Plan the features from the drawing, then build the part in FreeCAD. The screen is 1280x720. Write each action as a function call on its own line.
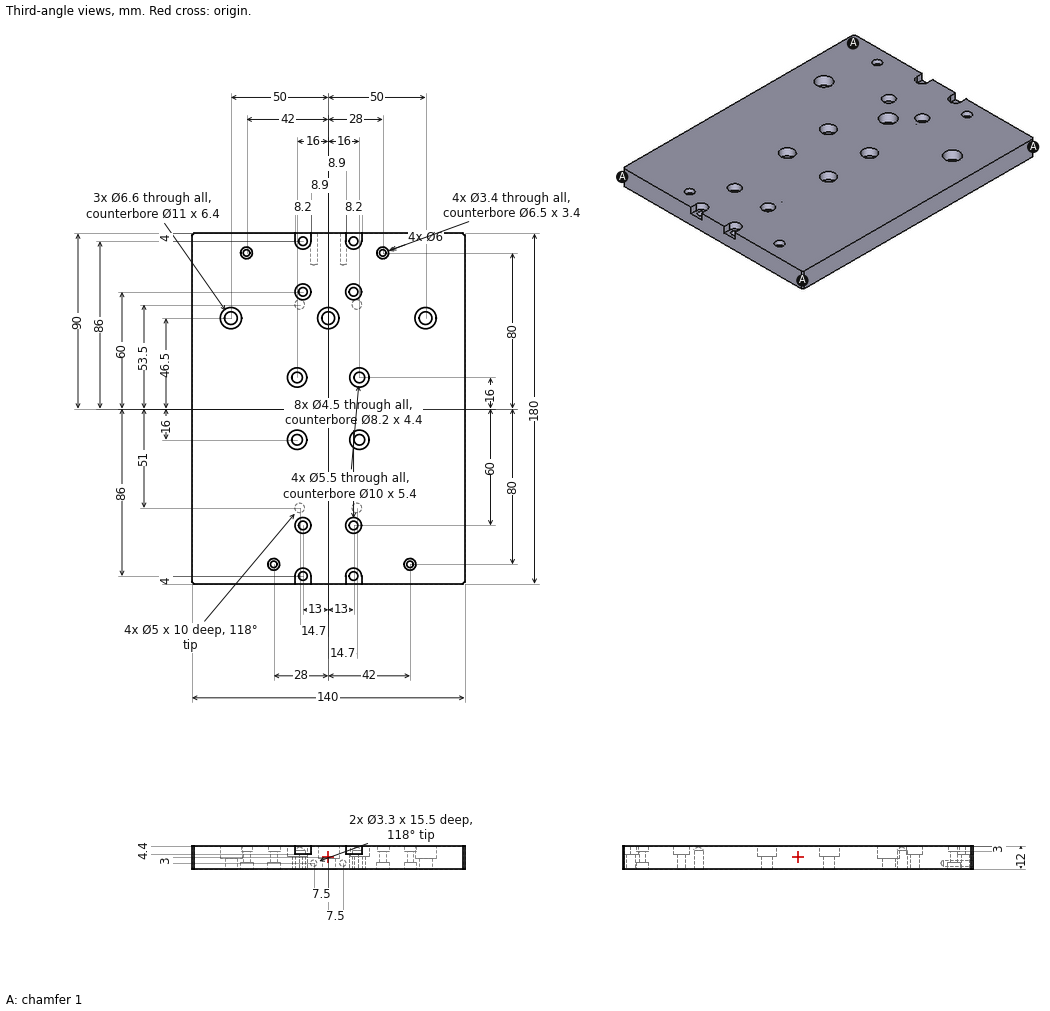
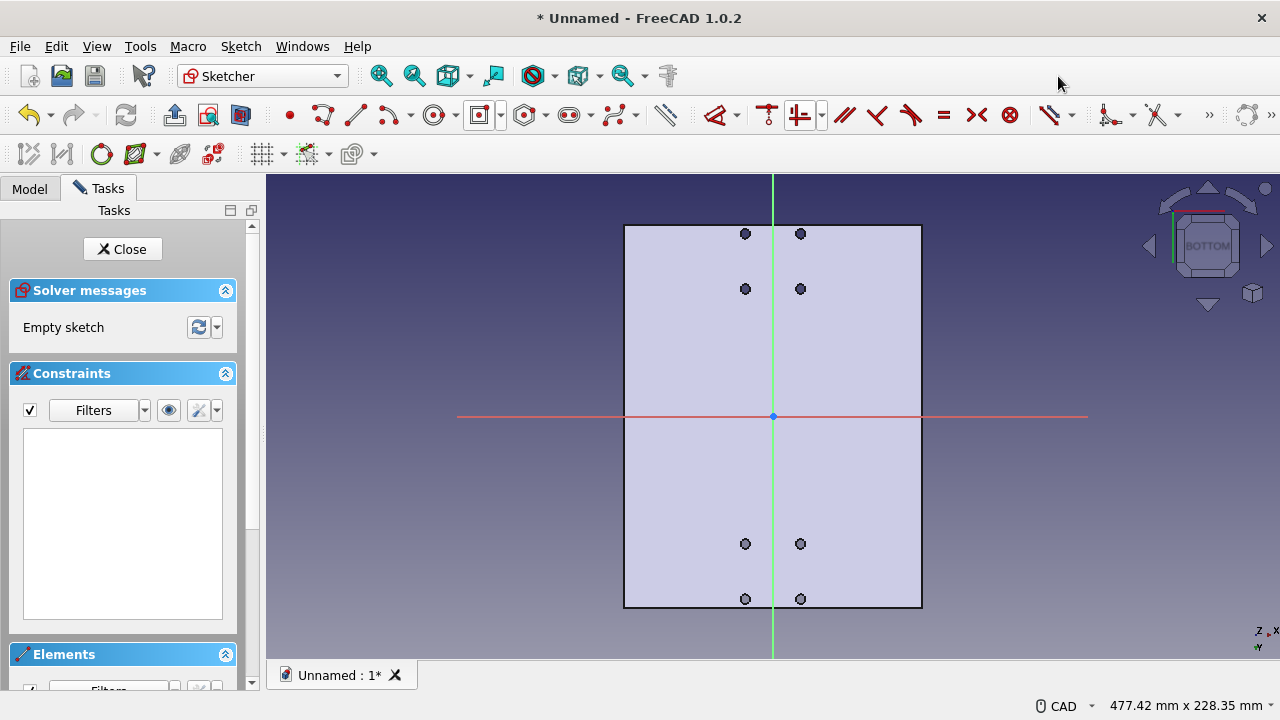
click(434, 116)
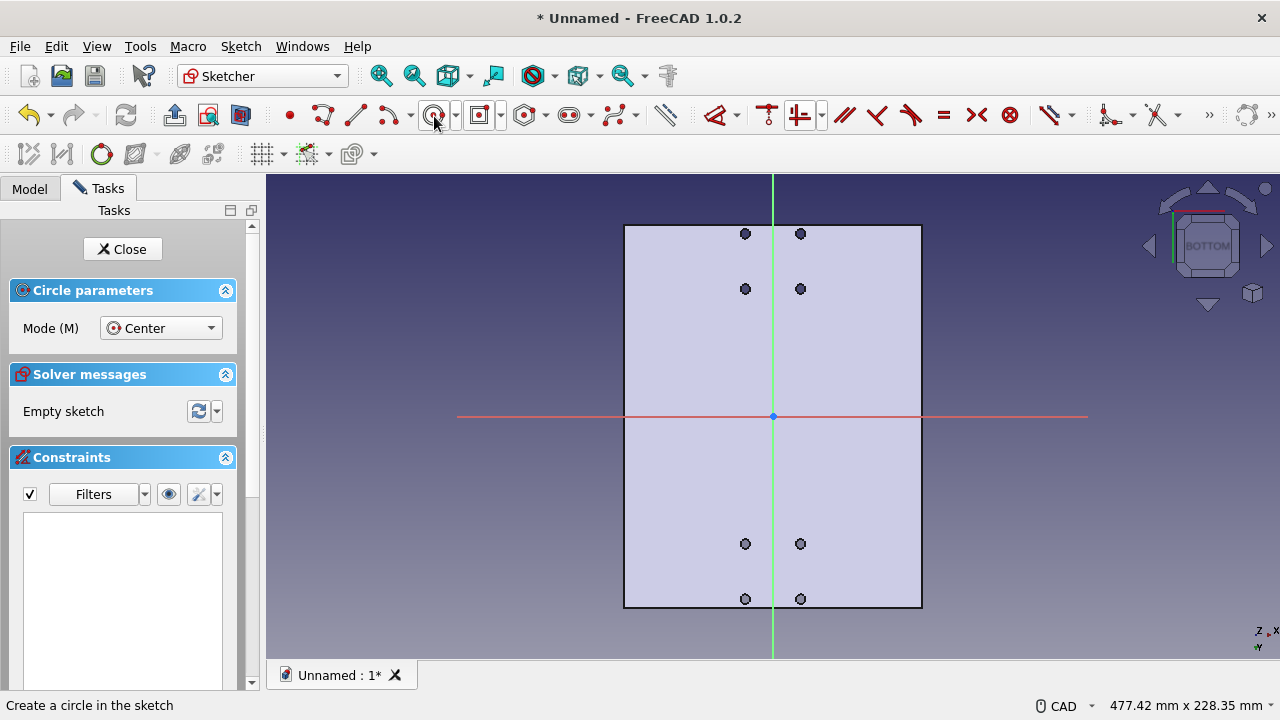
scroll(742, 308, up, 8)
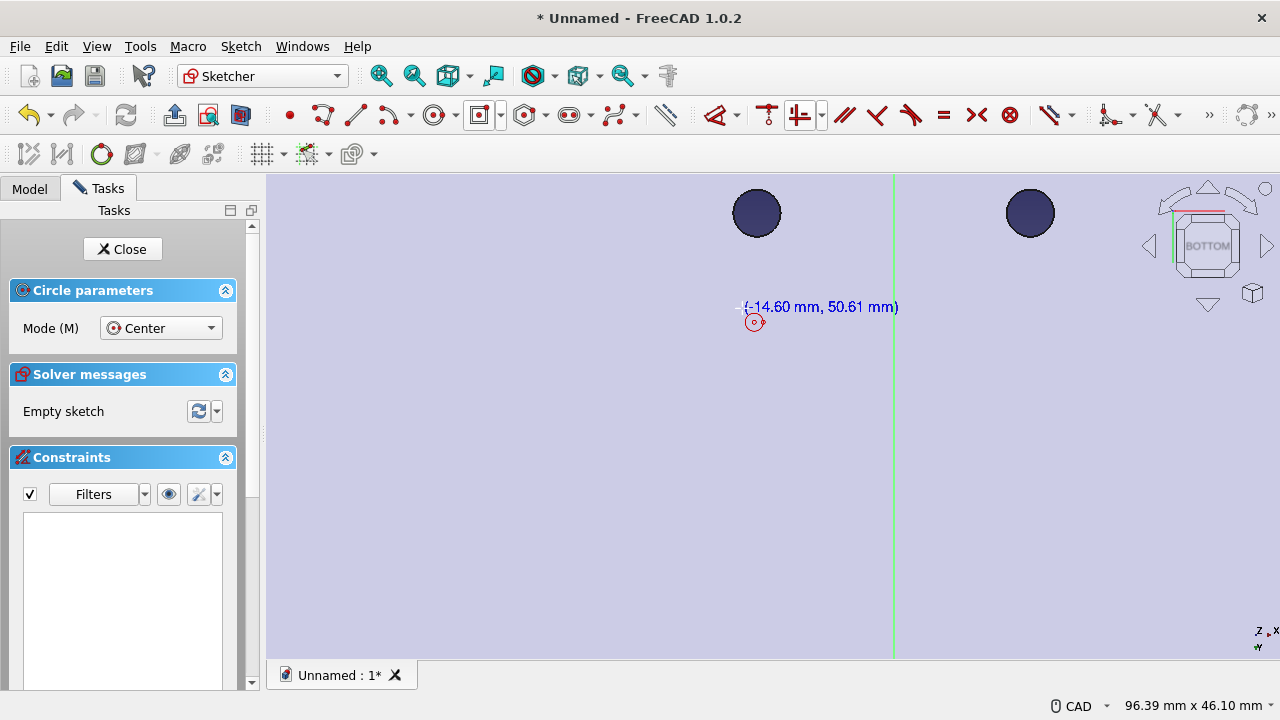
scroll(643, 272, down, 7)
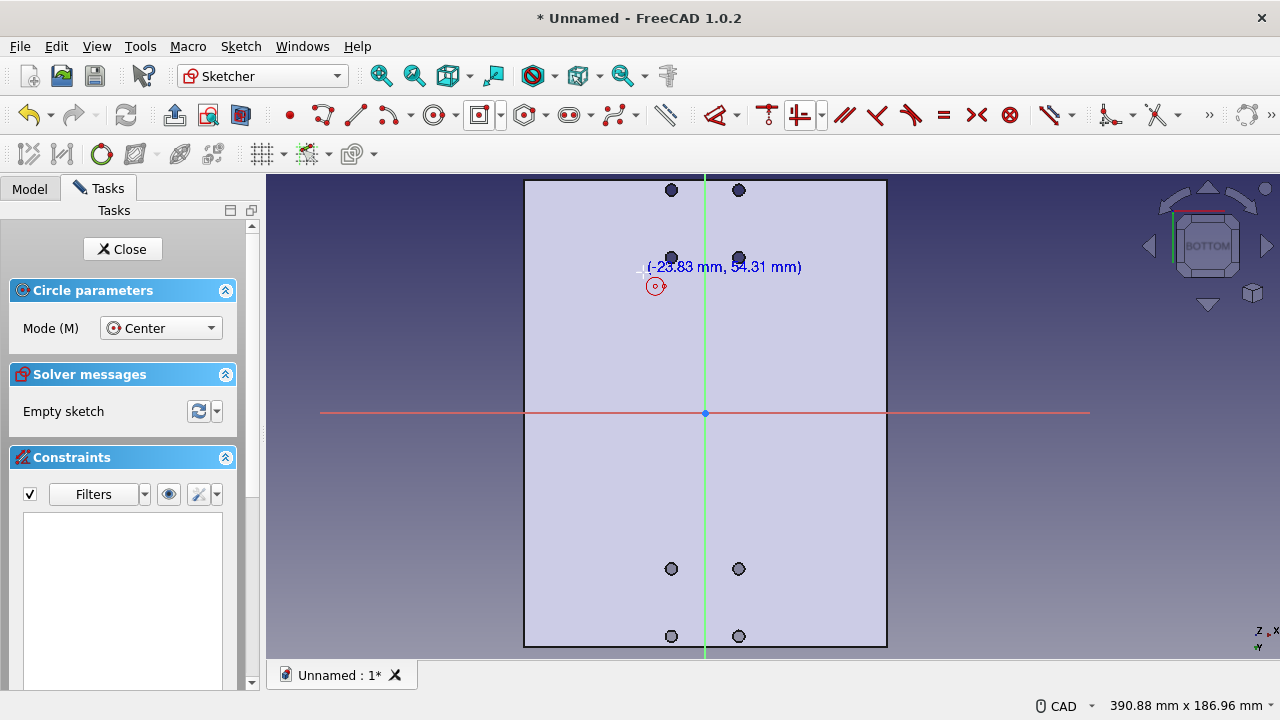
click(667, 281)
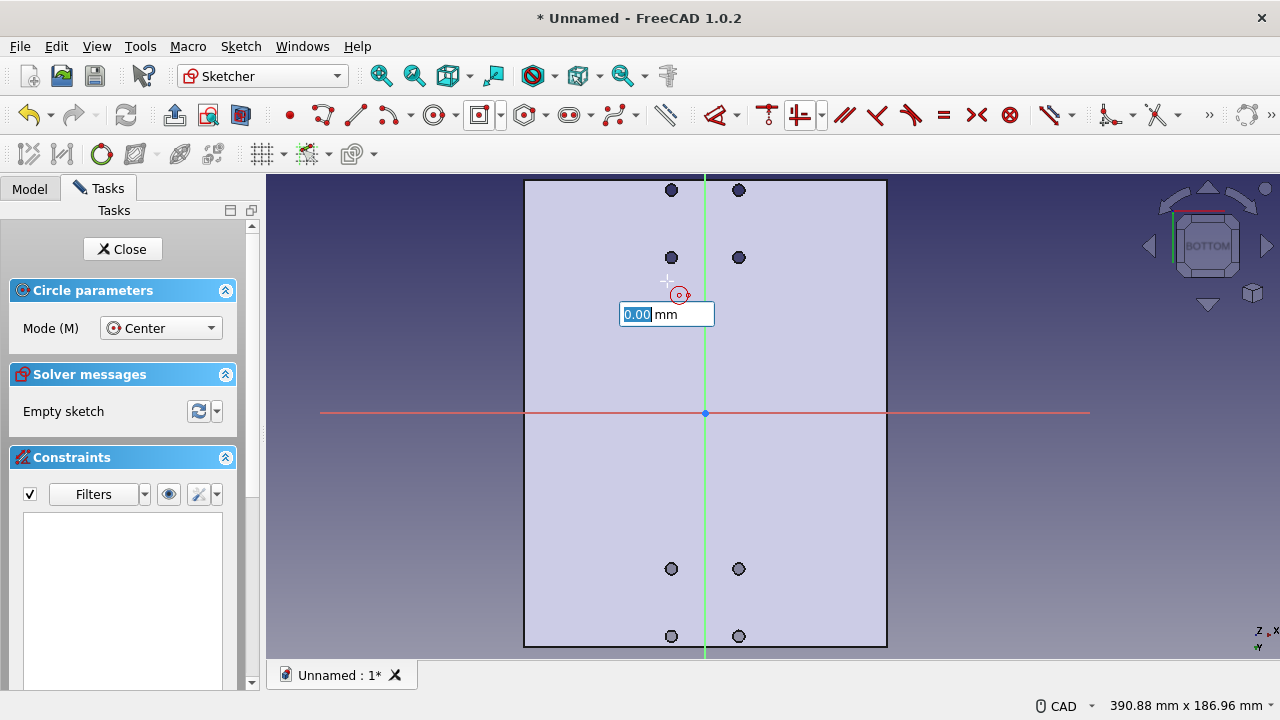
scroll(672, 276, up, 5)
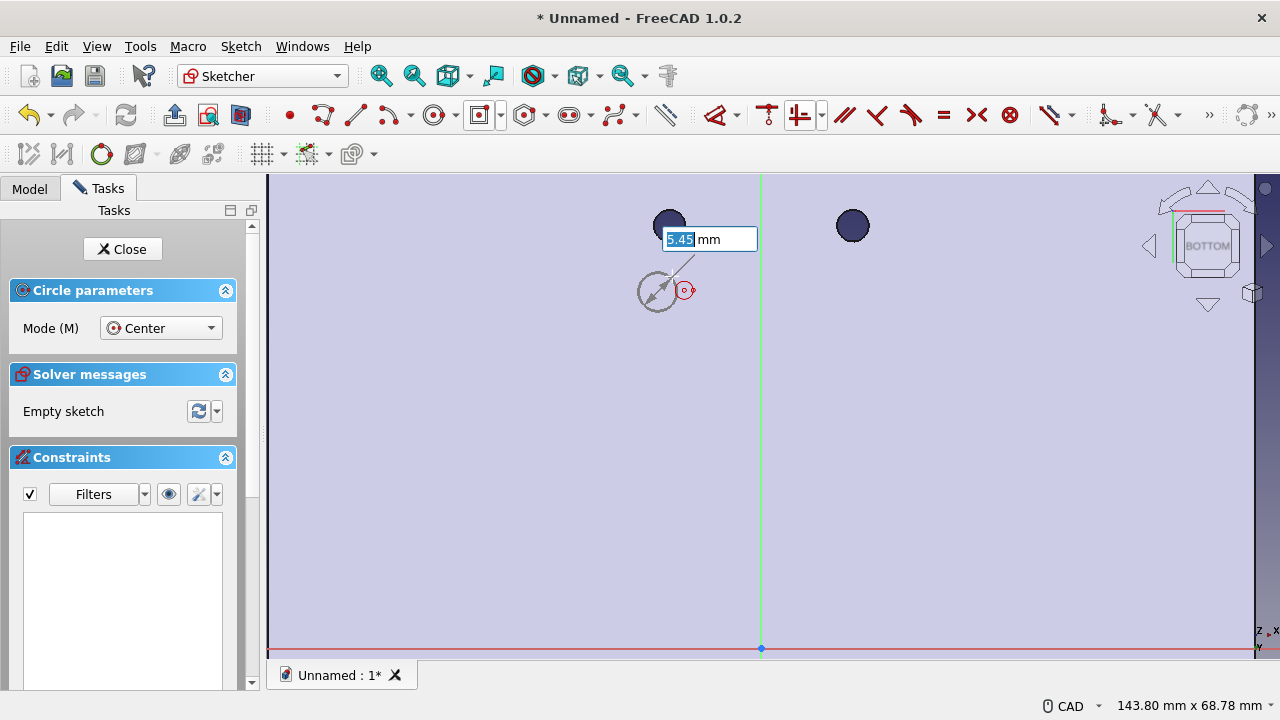
click(670, 277)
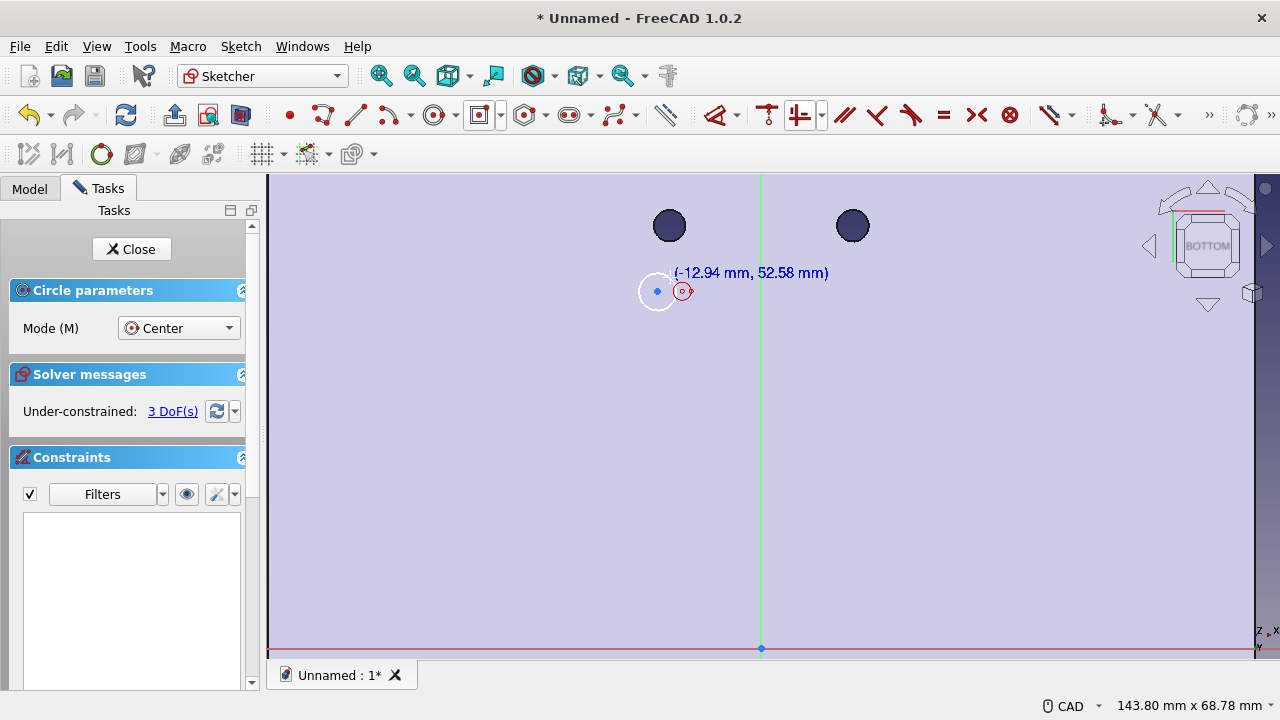
scroll(865, 289, up, 2)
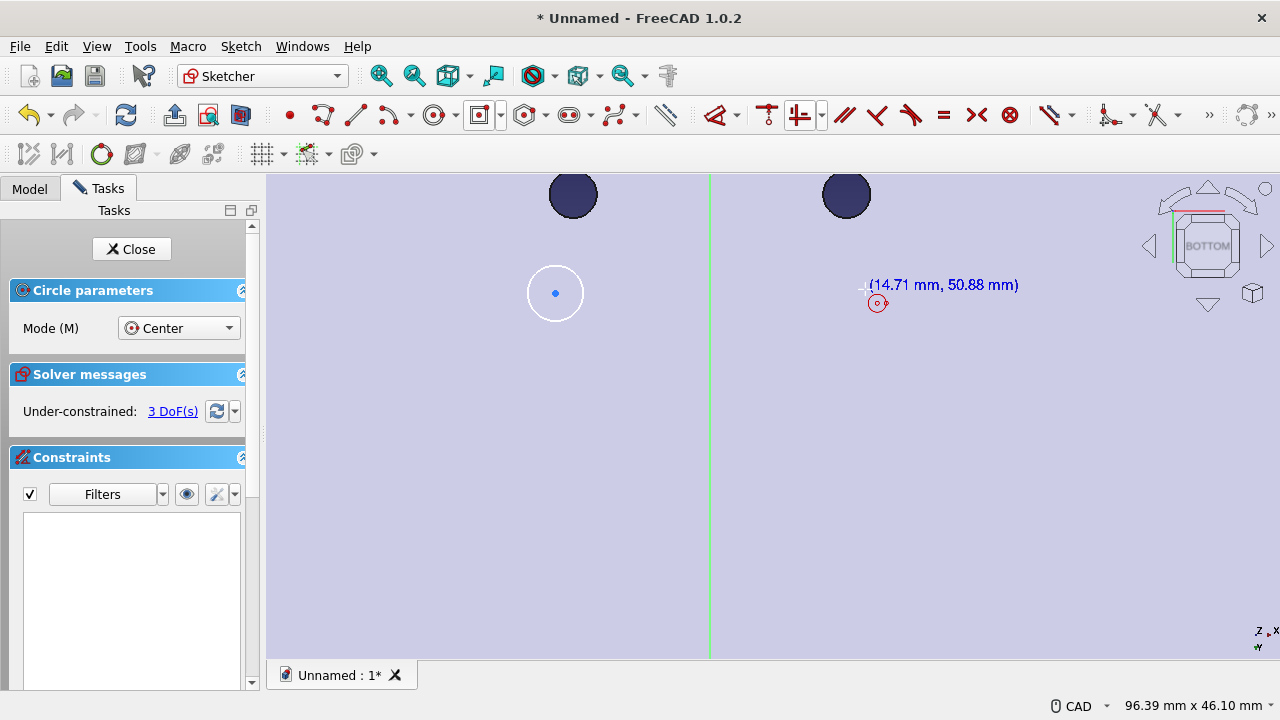
scroll(703, 278, down, 7)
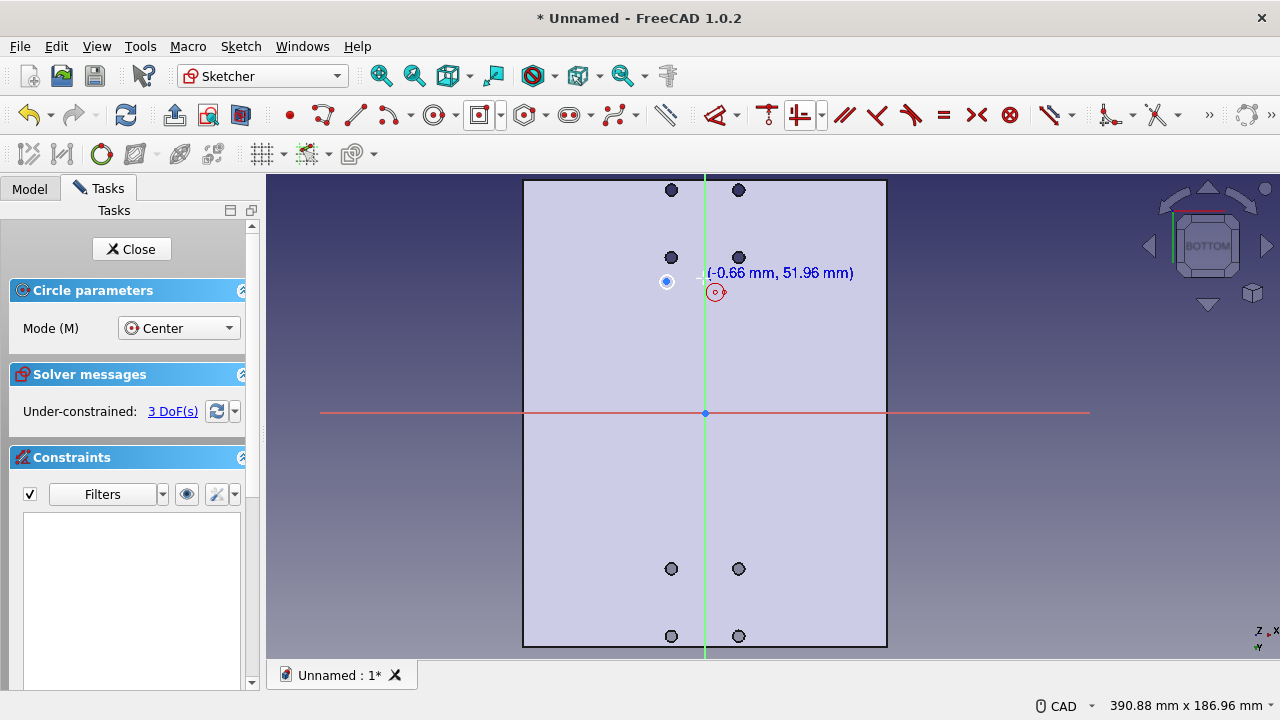
click(743, 281)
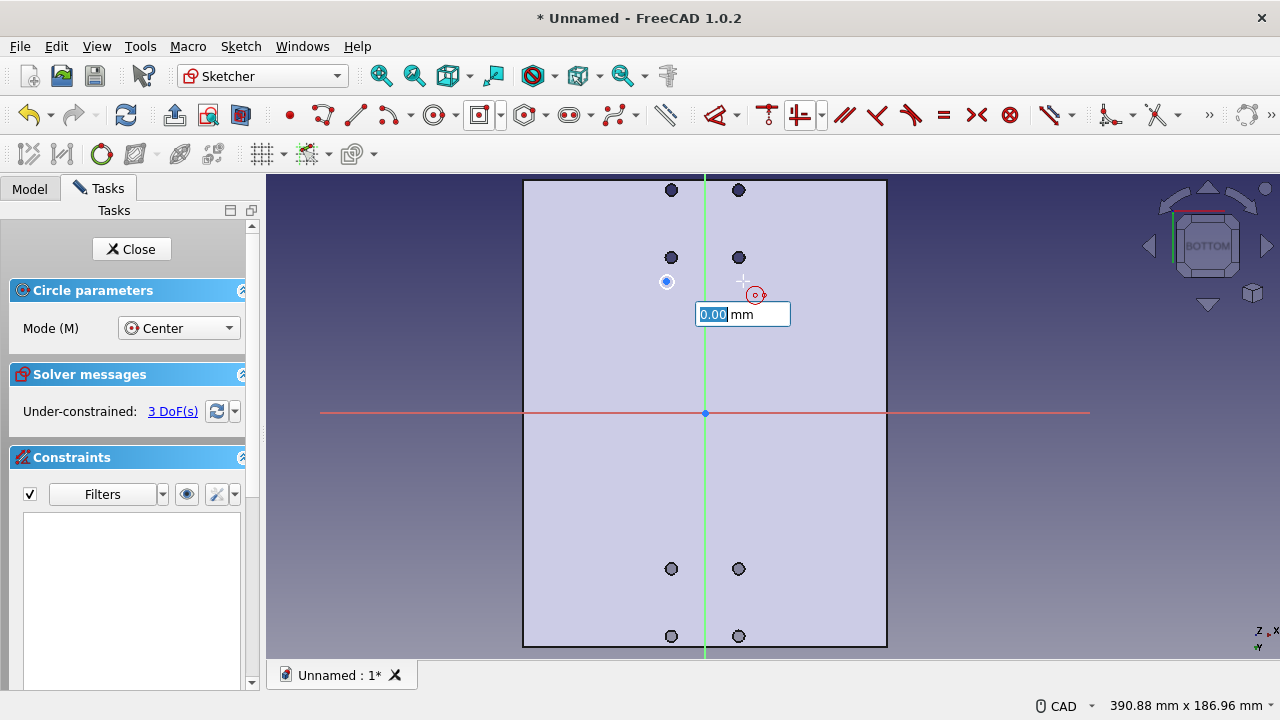
scroll(748, 276, up, 5)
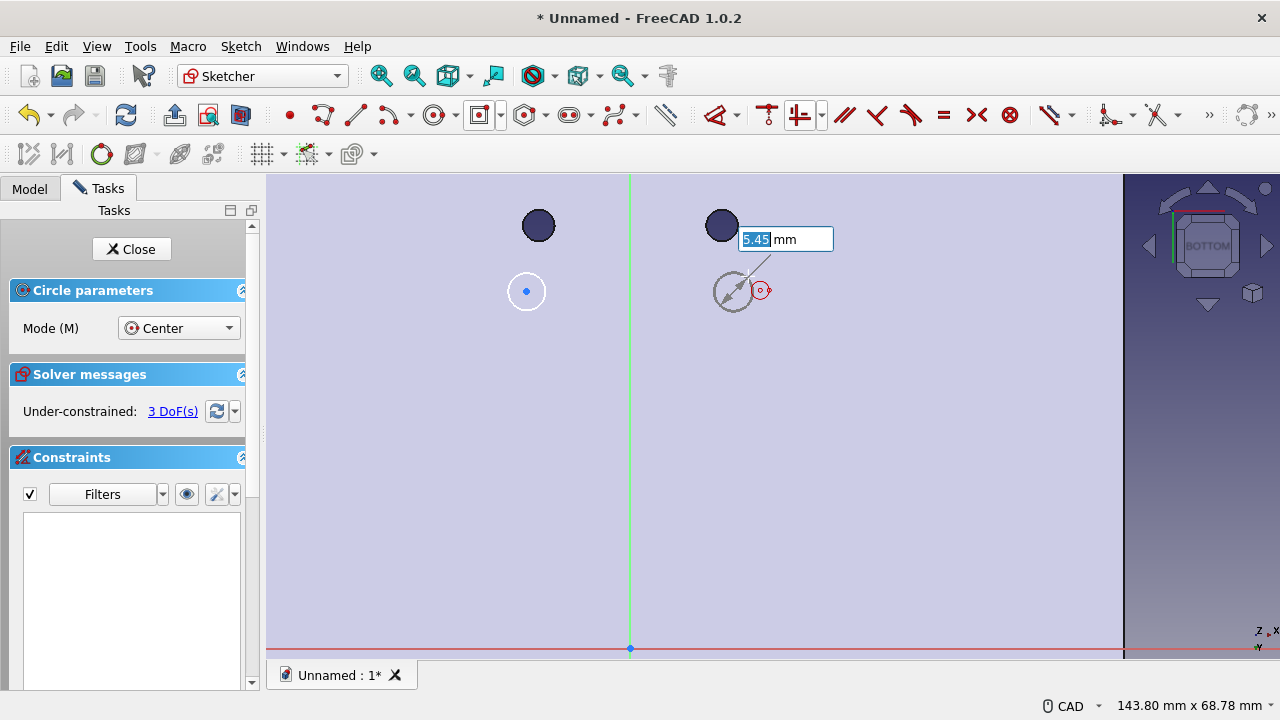
click(747, 277)